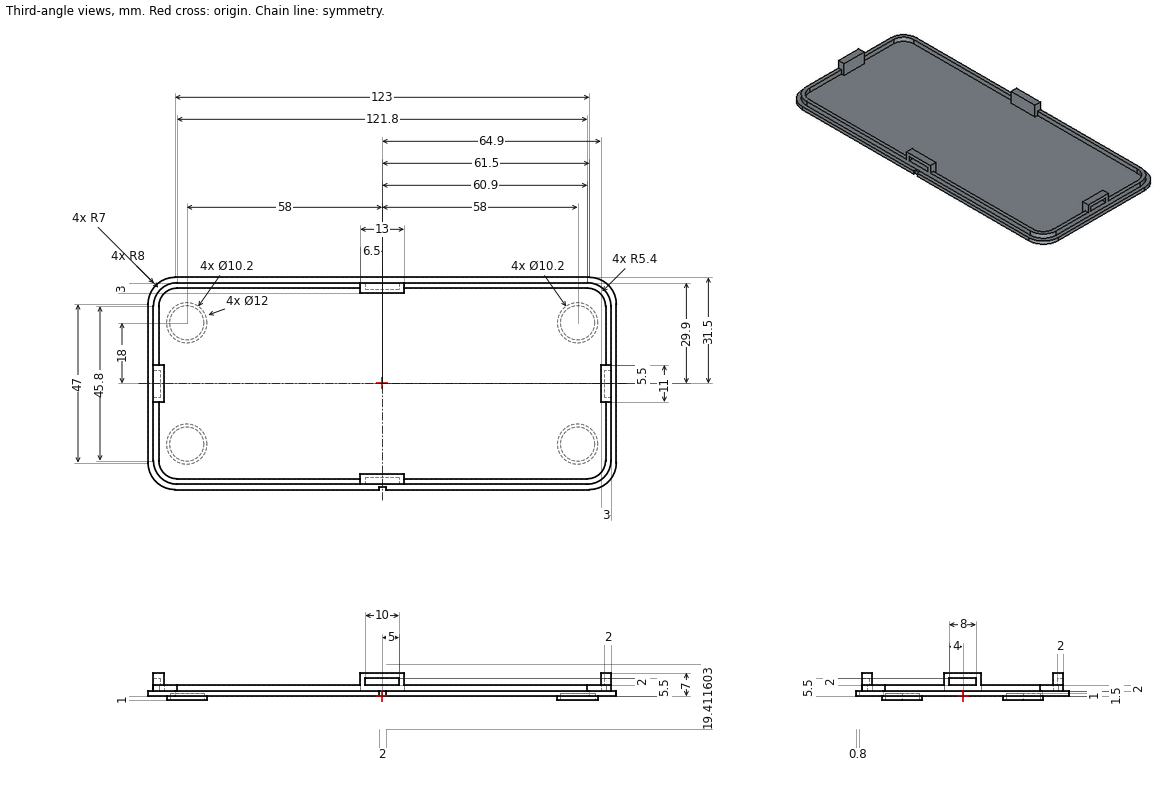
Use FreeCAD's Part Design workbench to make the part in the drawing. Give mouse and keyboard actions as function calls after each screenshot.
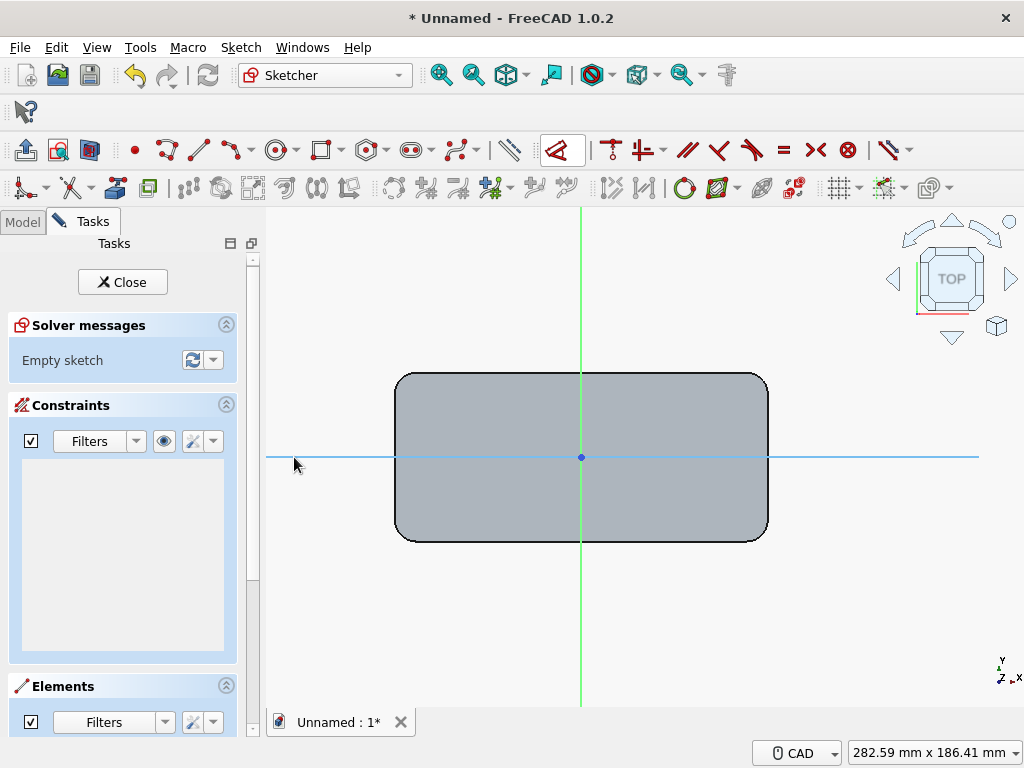
key(g)
key(l)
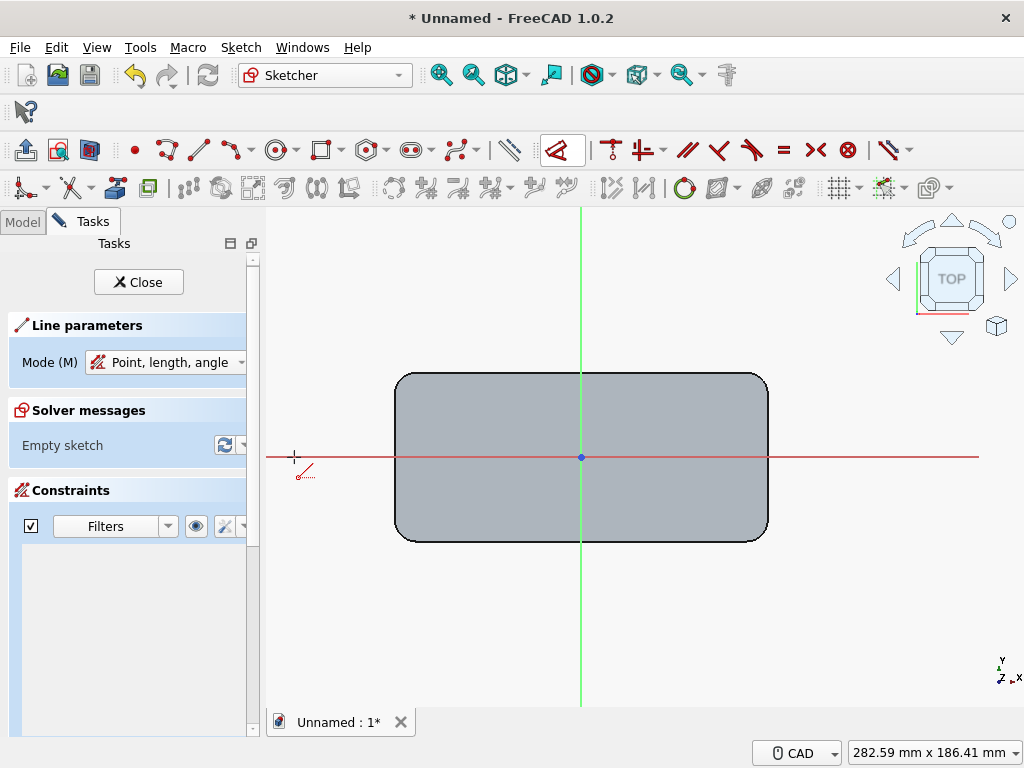
click(745, 377)
click(418, 377)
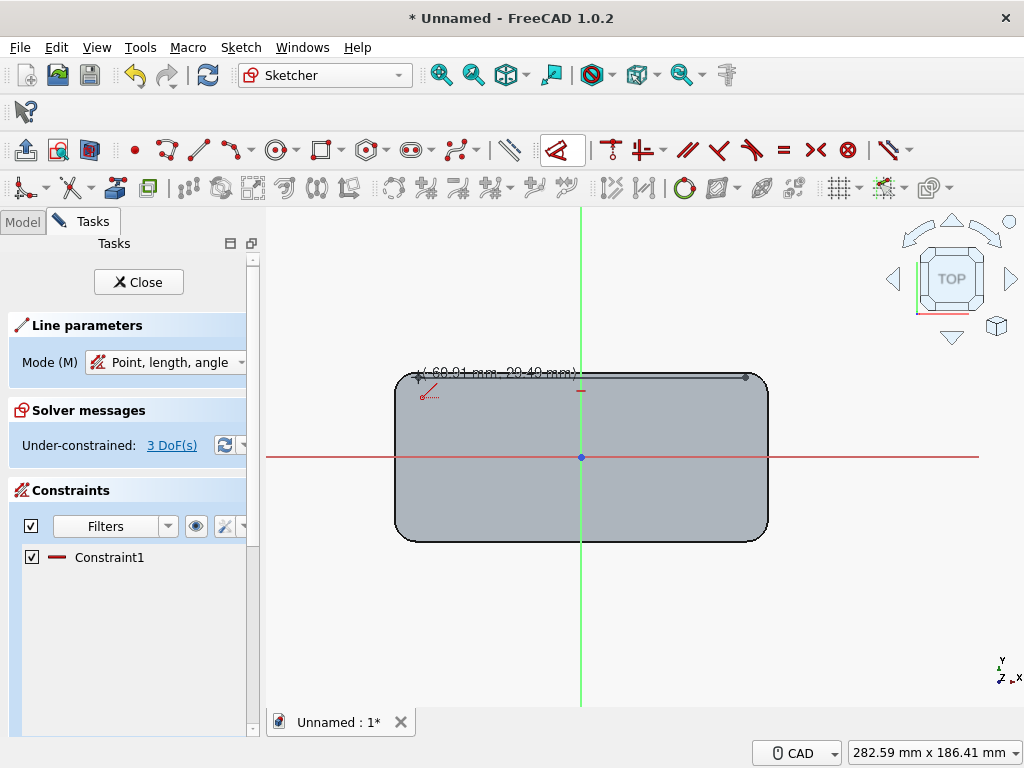
click(399, 396)
click(399, 519)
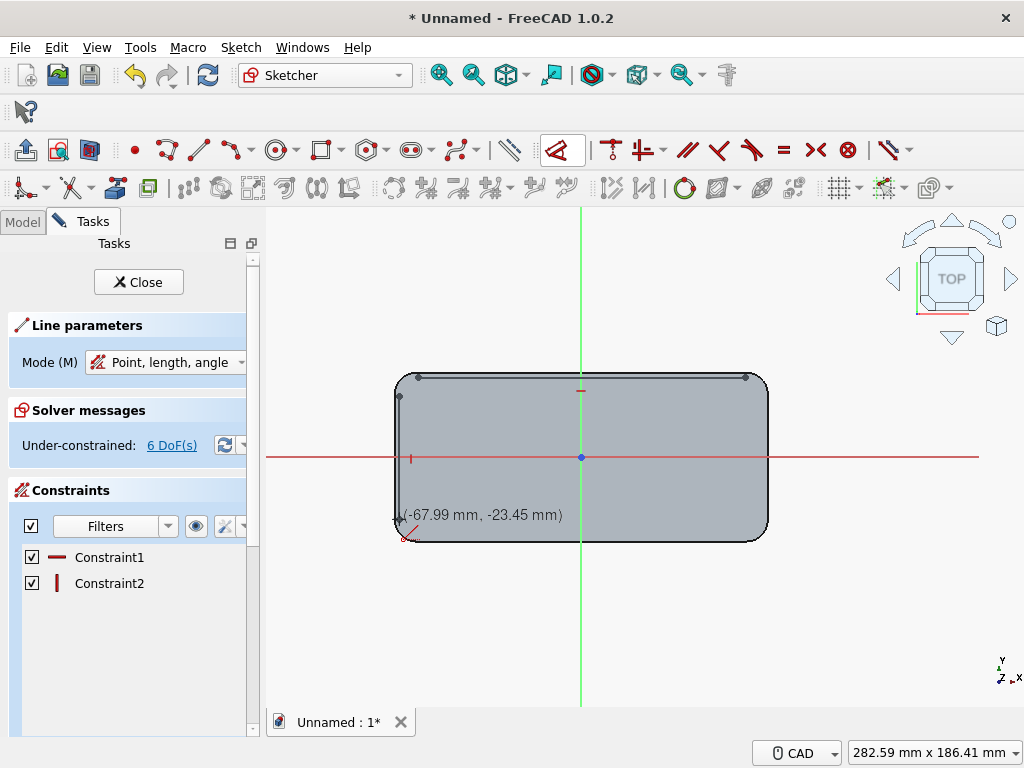
click(418, 537)
click(745, 537)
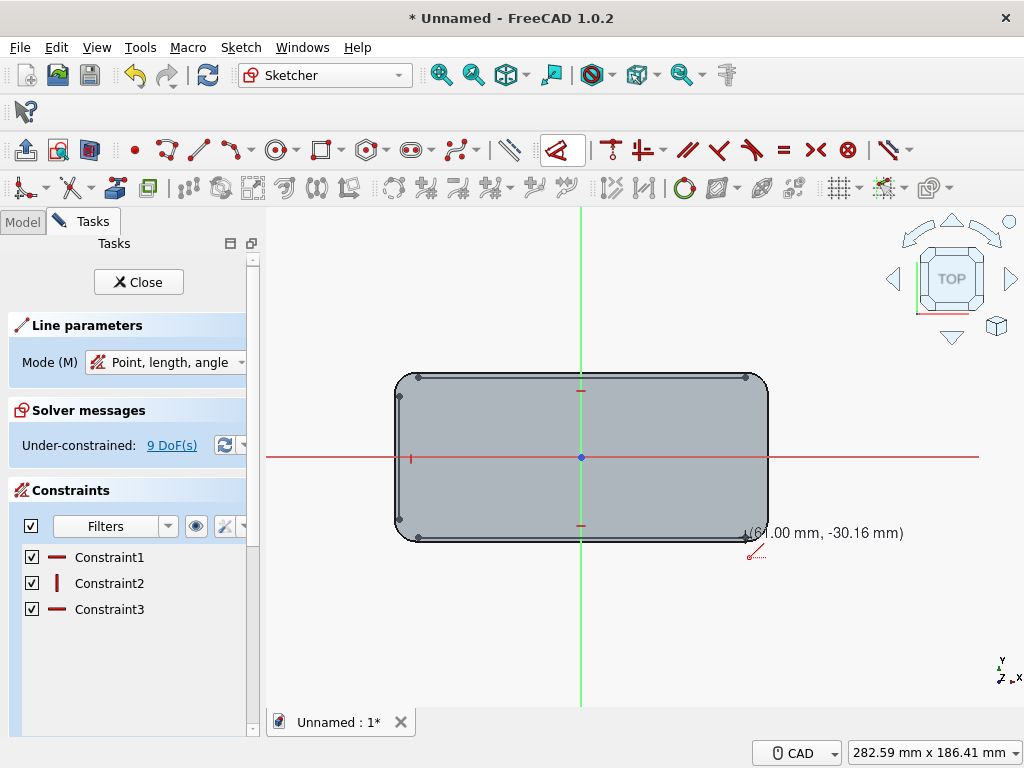
click(764, 519)
click(764, 396)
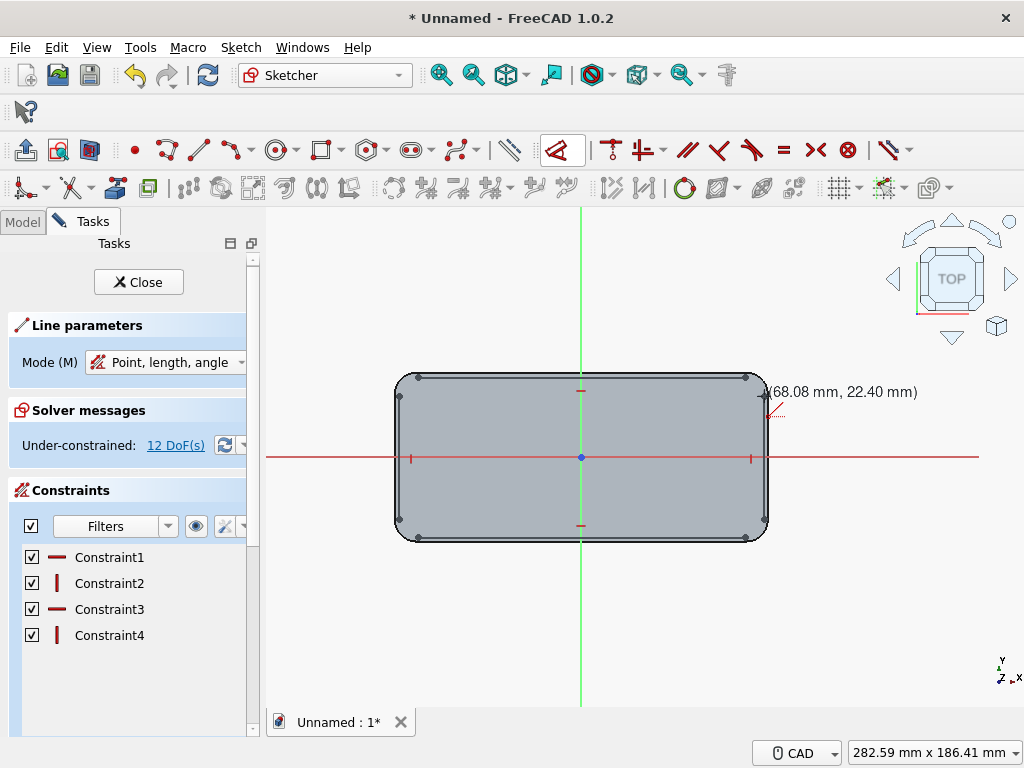
click(232, 150)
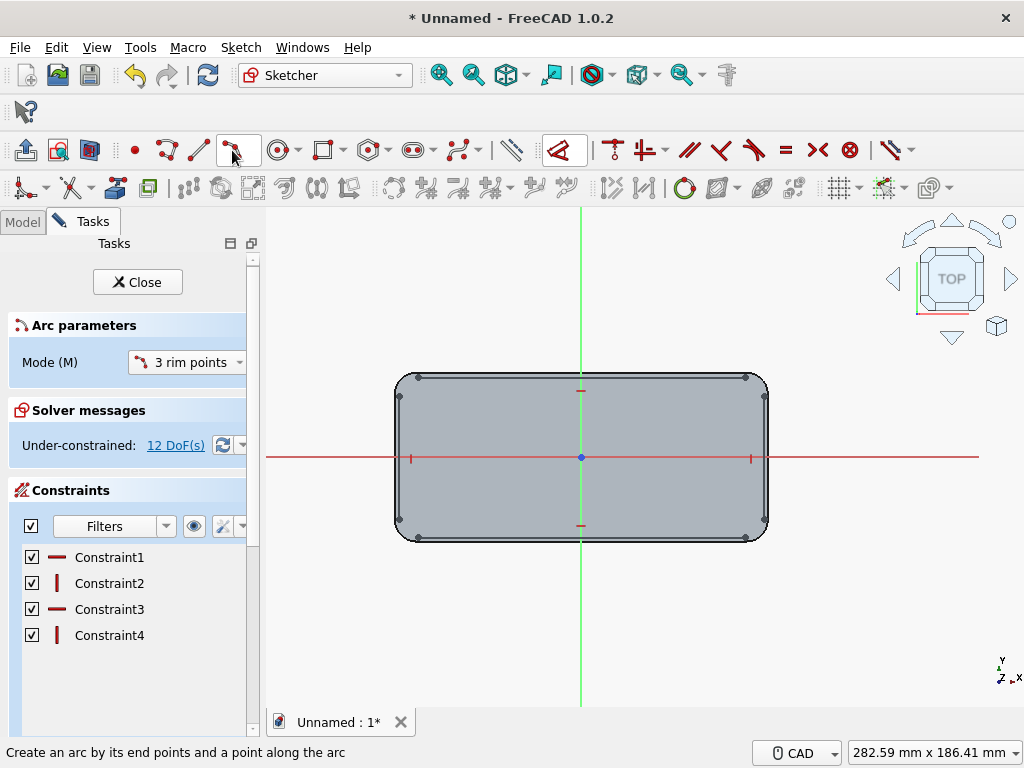
click(418, 378)
click(399, 397)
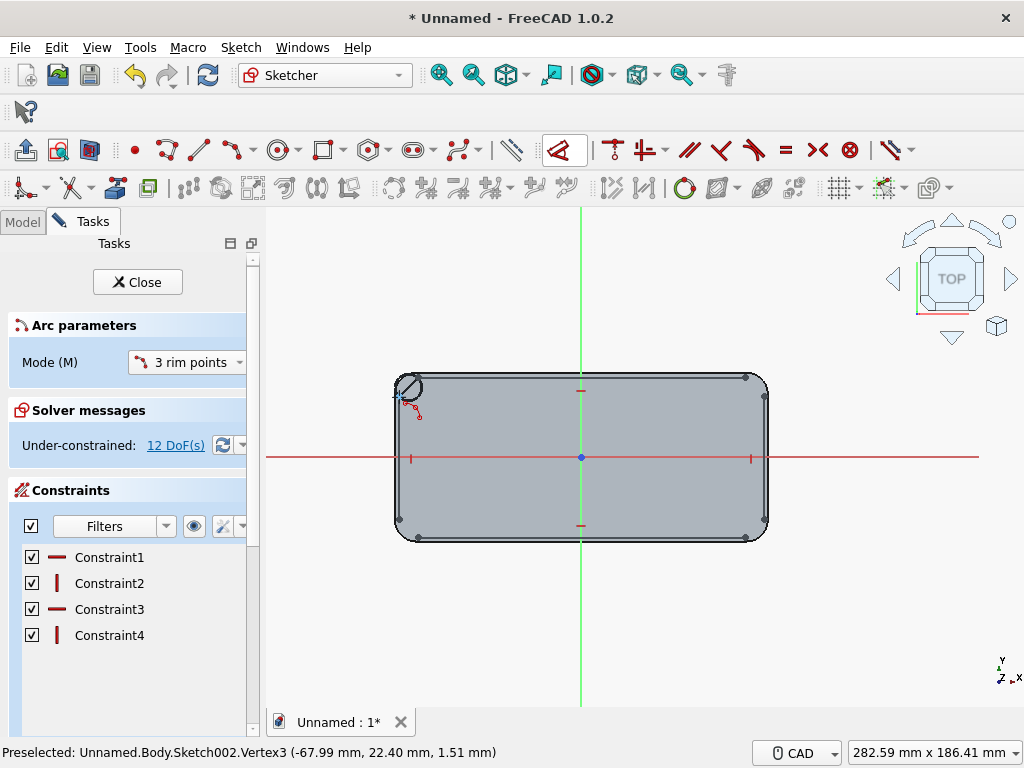
scroll(405, 382, up, 6)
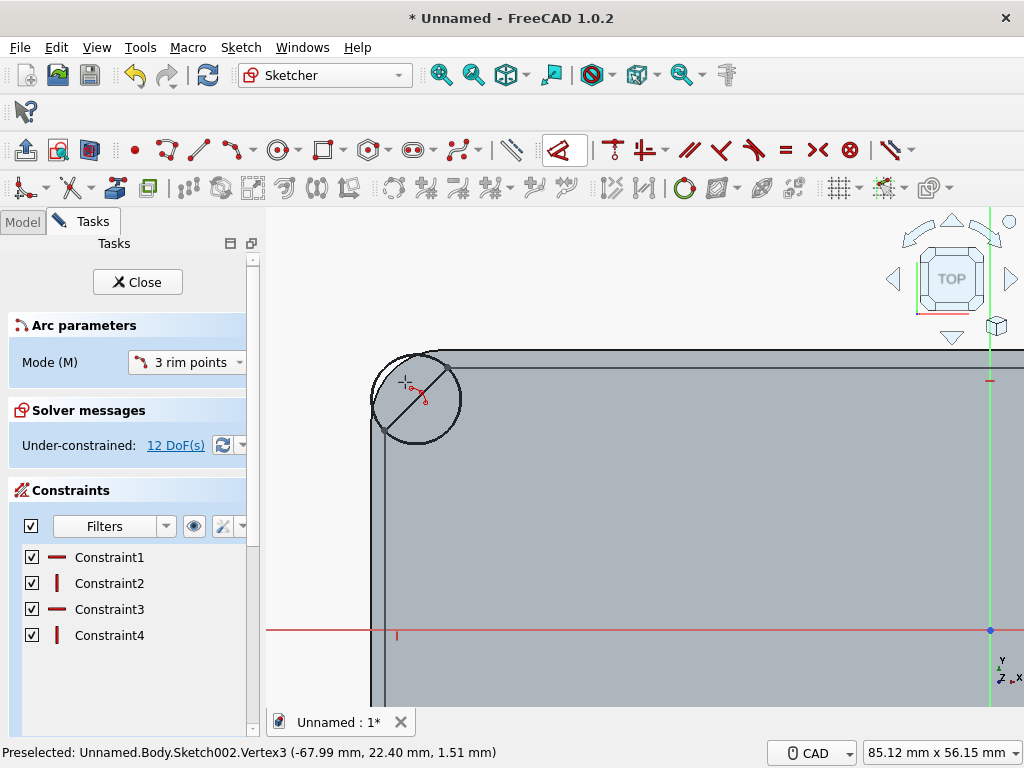
click(404, 382)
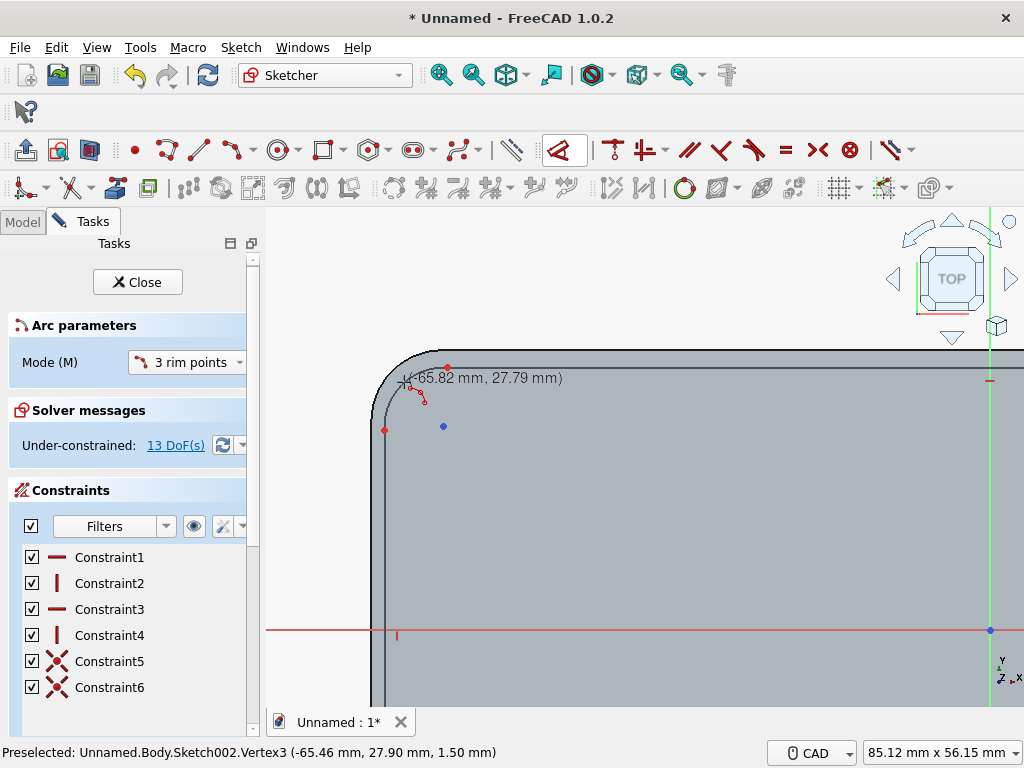
scroll(398, 382, down, 6)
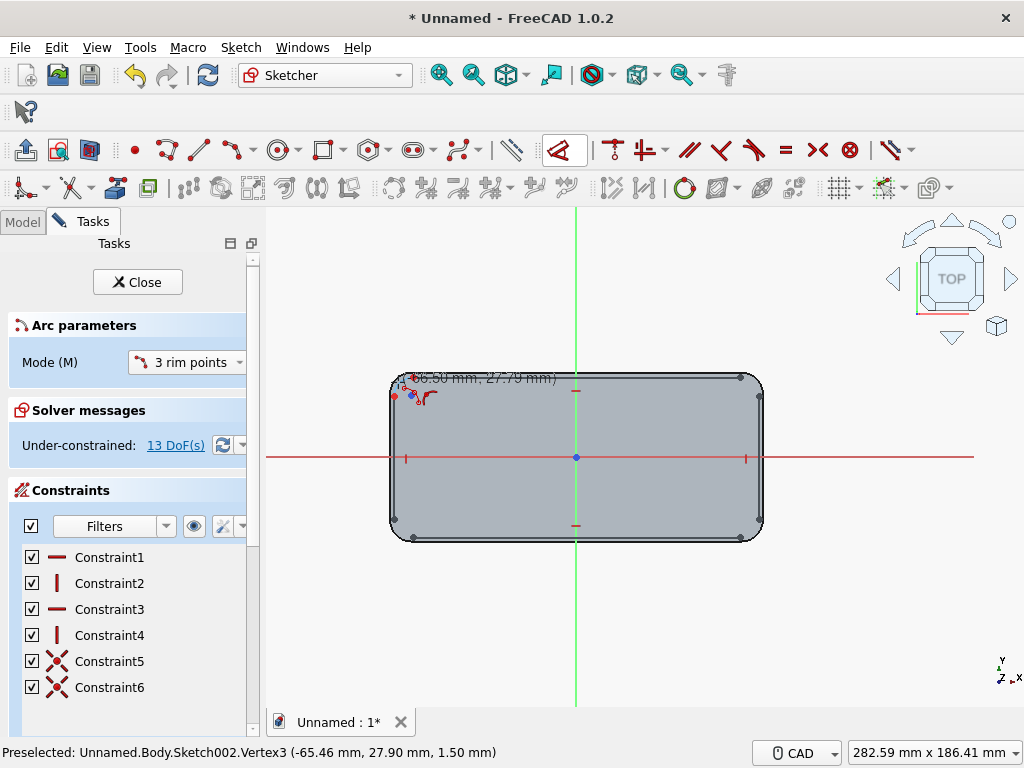
click(394, 520)
click(413, 538)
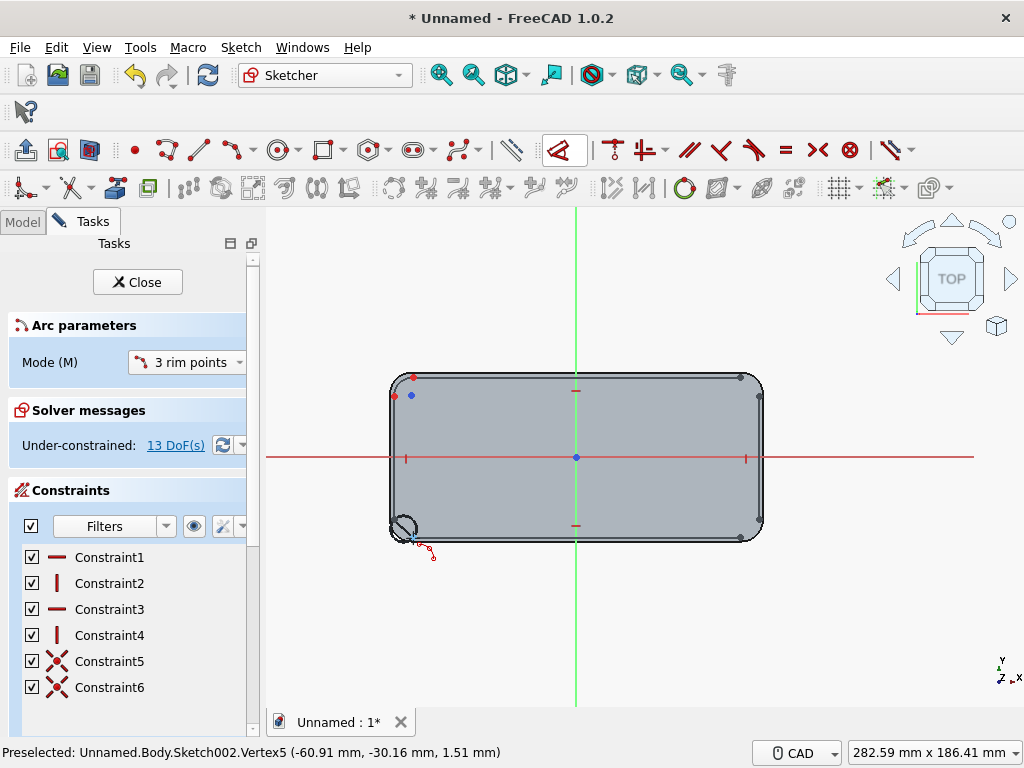
scroll(400, 532, up, 6)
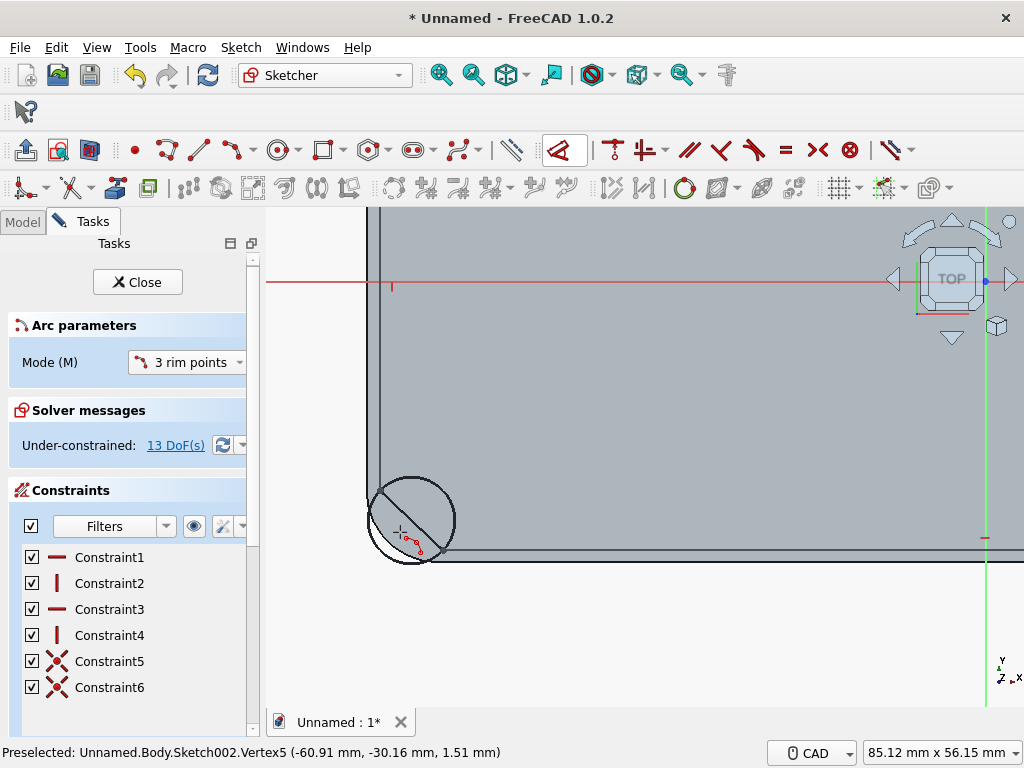
click(399, 530)